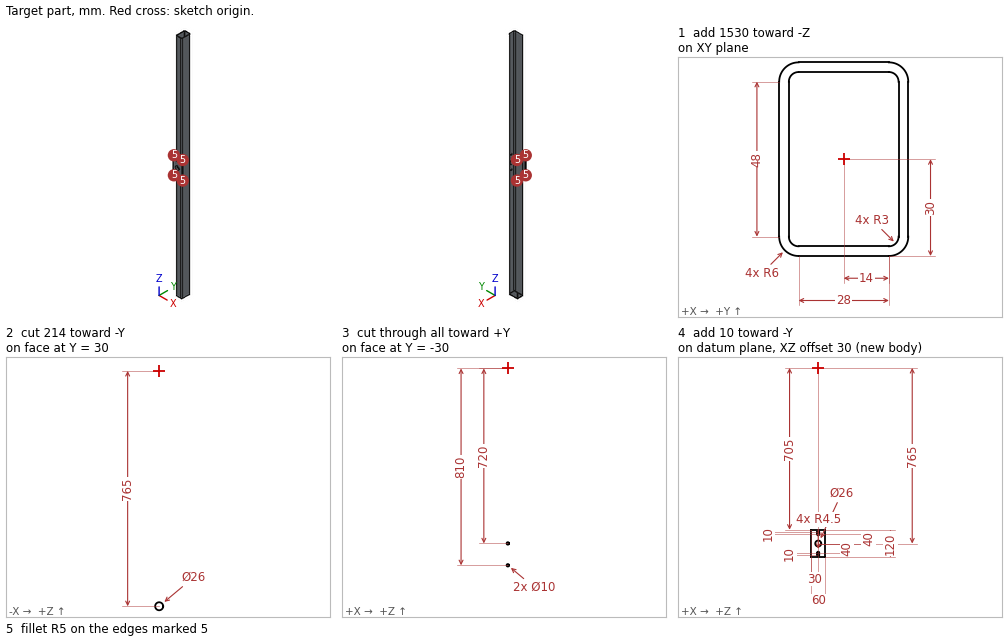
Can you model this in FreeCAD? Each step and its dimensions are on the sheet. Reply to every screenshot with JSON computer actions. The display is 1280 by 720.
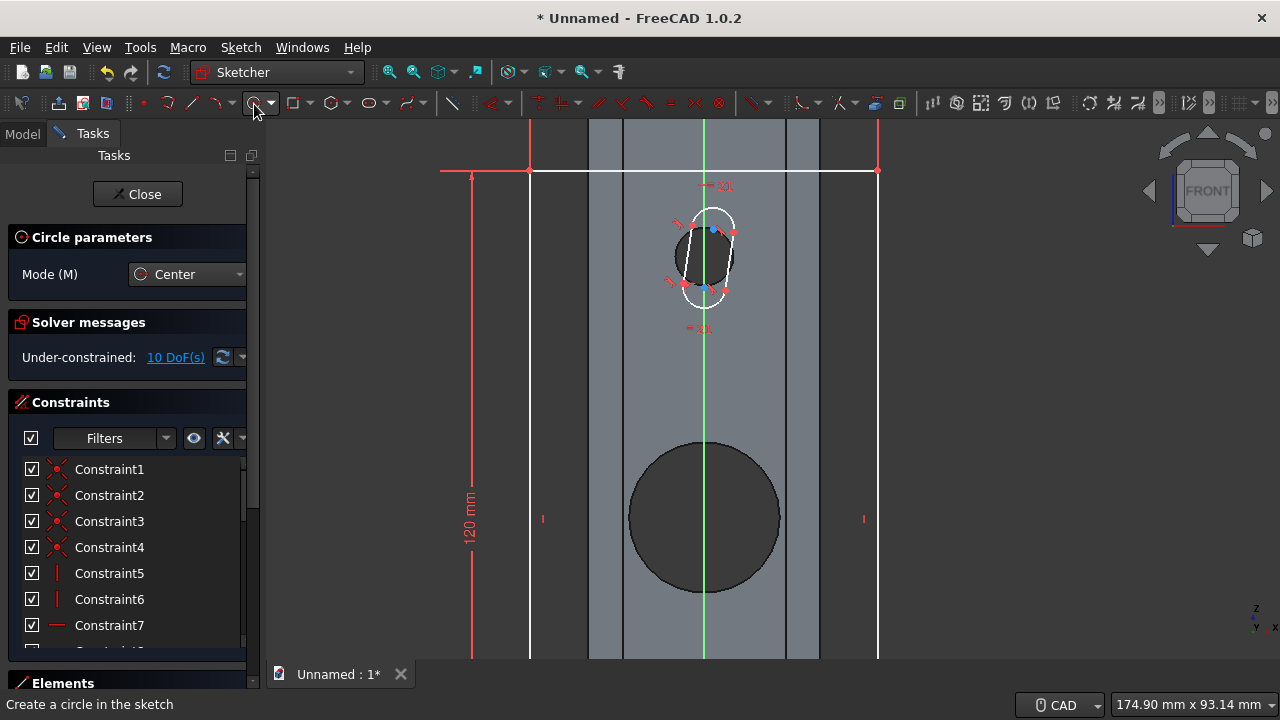
{"action": "left_click", "coordinate": [704, 518]}
{"action": "mouse_move", "coordinate": [758, 464]}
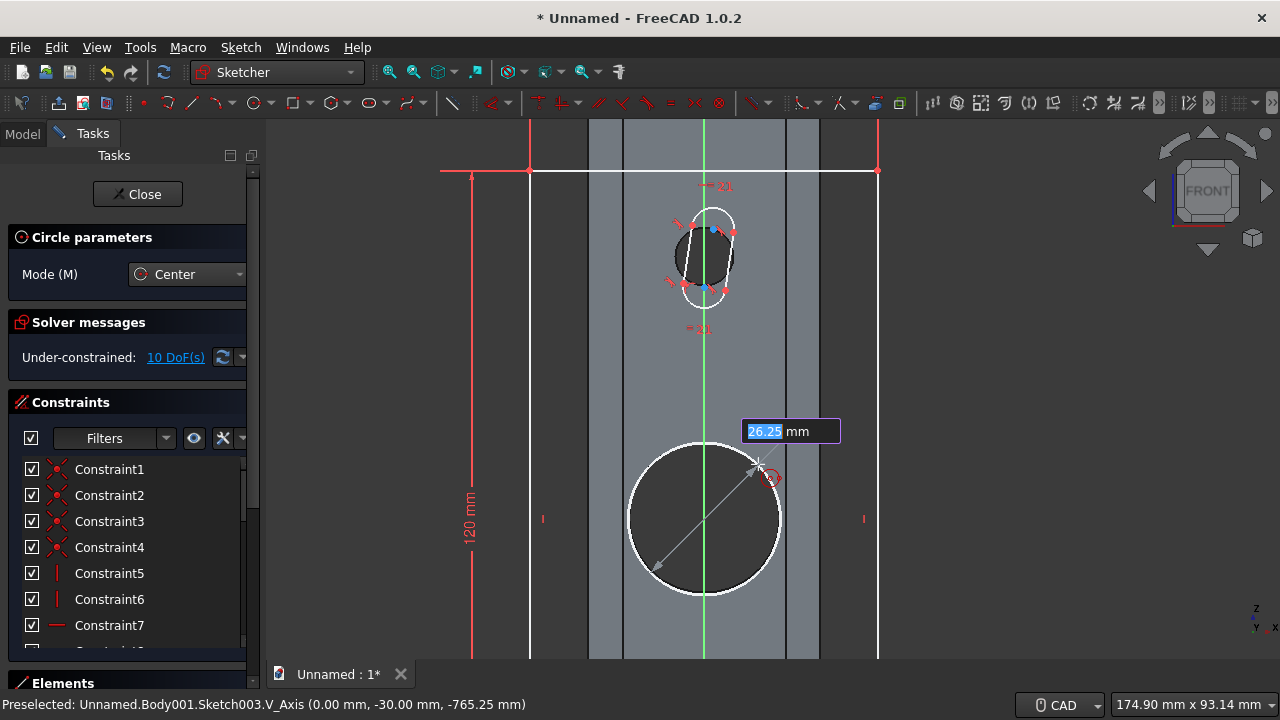
{"action": "type", "text": "26"}
{"action": "key", "text": "Return"}
{"action": "key", "text": "Escape"}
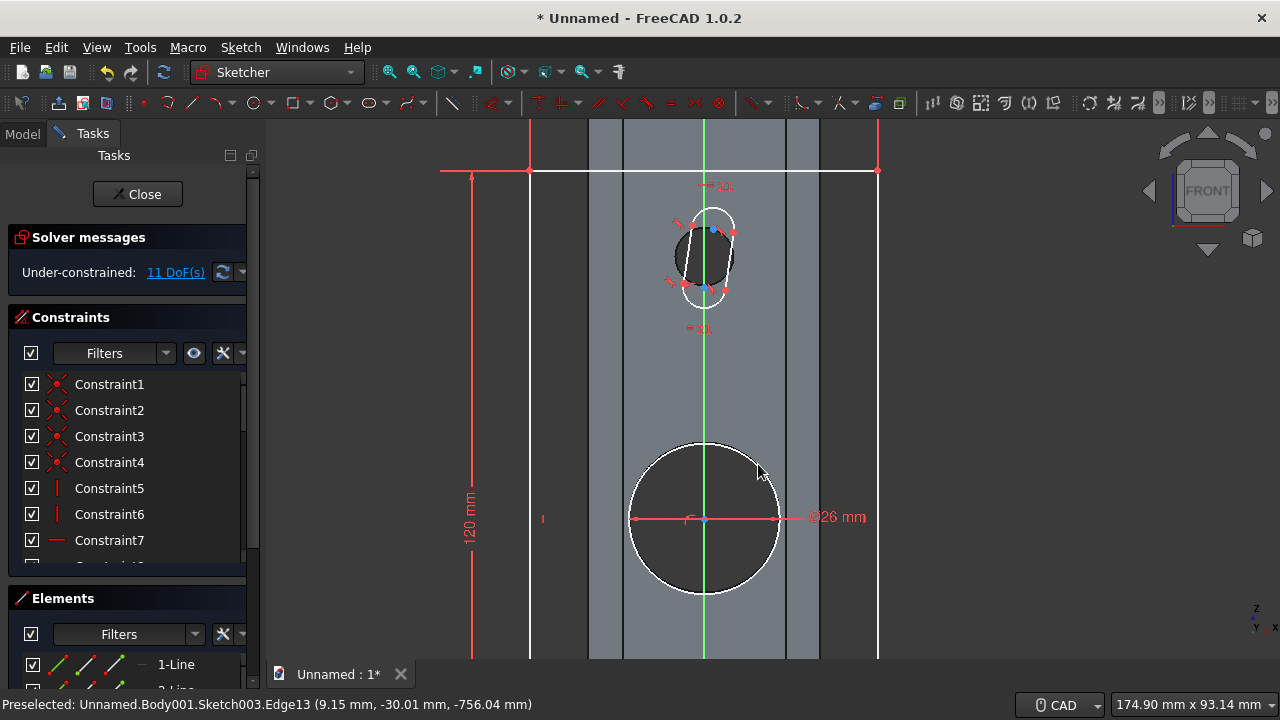
{"action": "scroll", "coordinate": [705, 284], "scroll_direction": "down", "scroll_amount": 4}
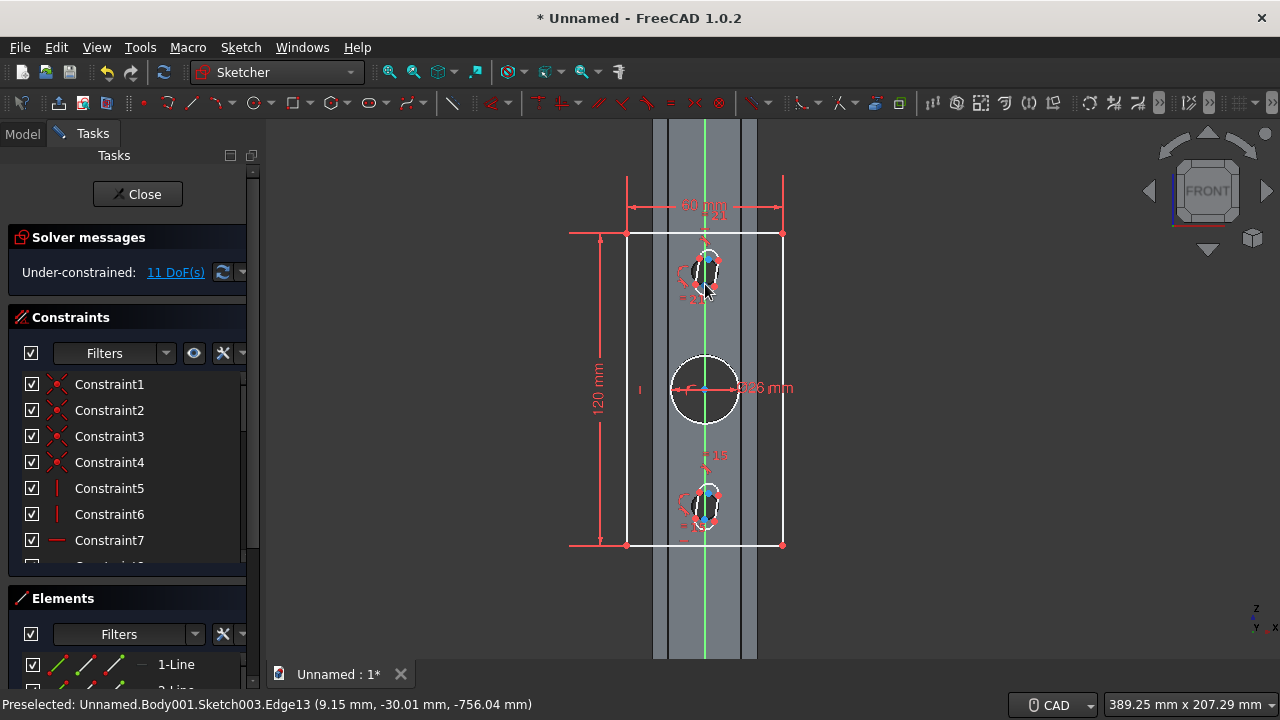
{"action": "scroll", "coordinate": [696, 510], "scroll_direction": "up", "scroll_amount": 3}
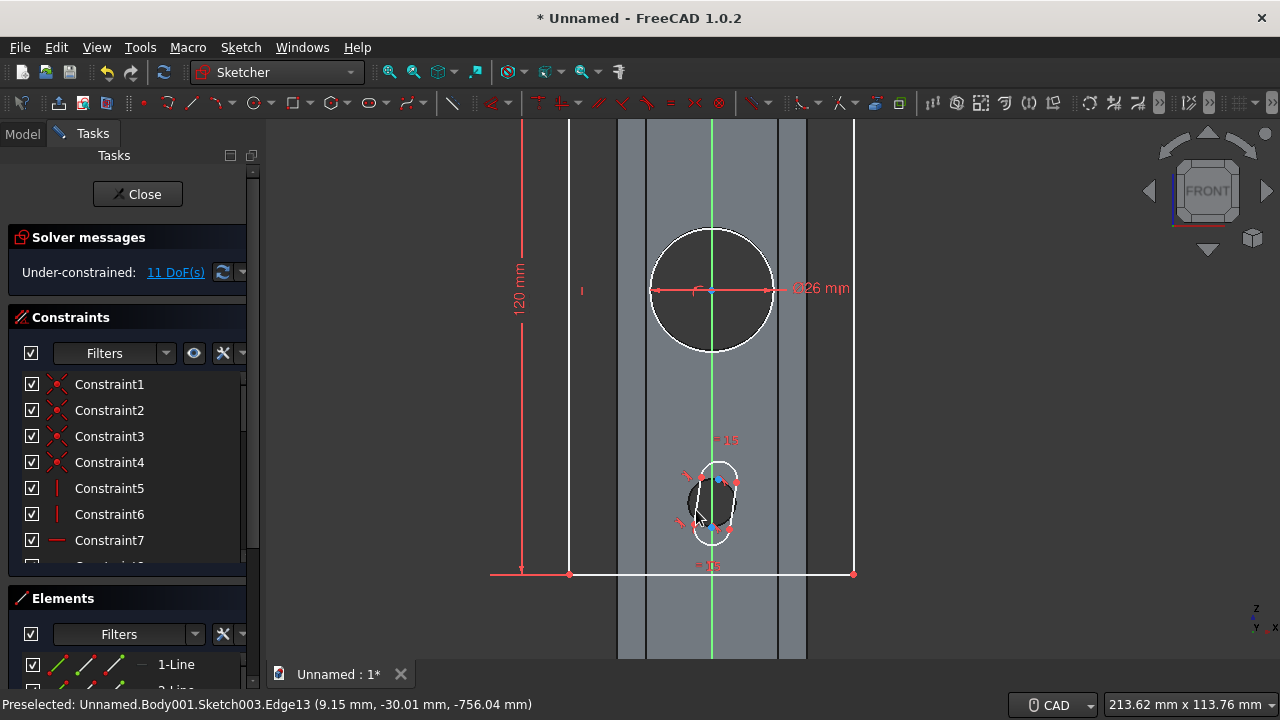
{"action": "left_click", "coordinate": [696, 510]}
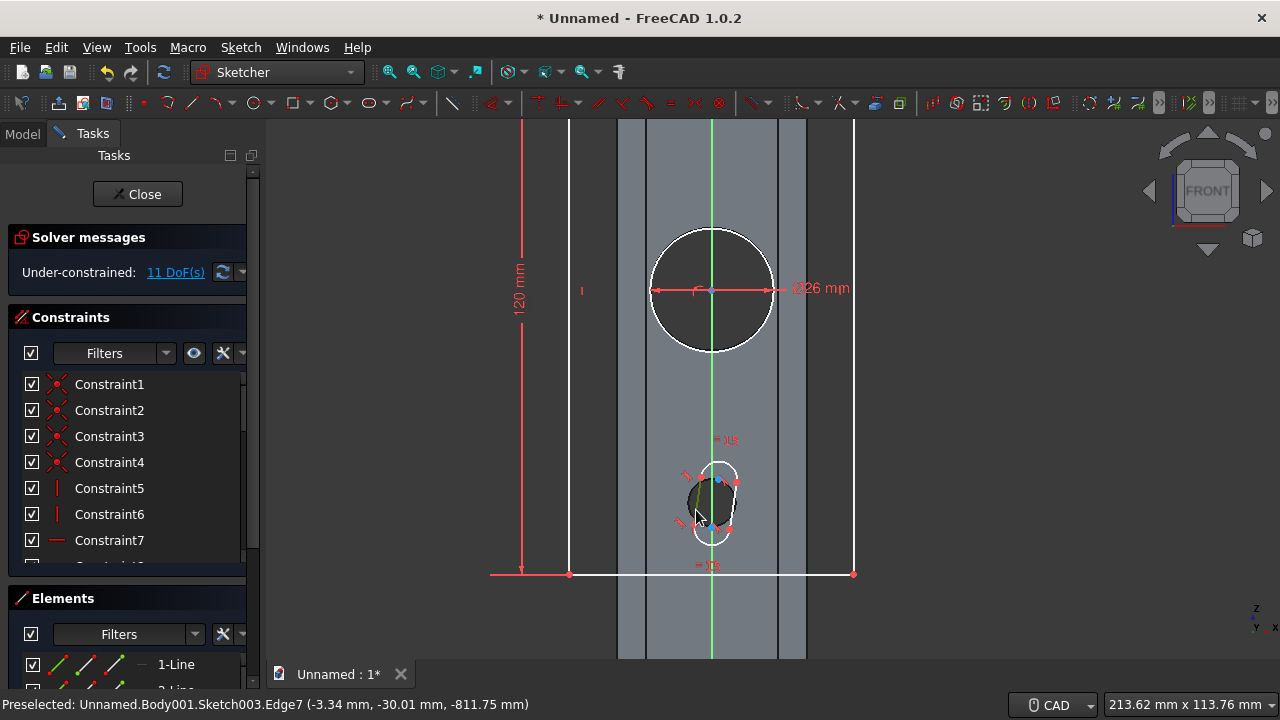
{"action": "key", "text": "v"}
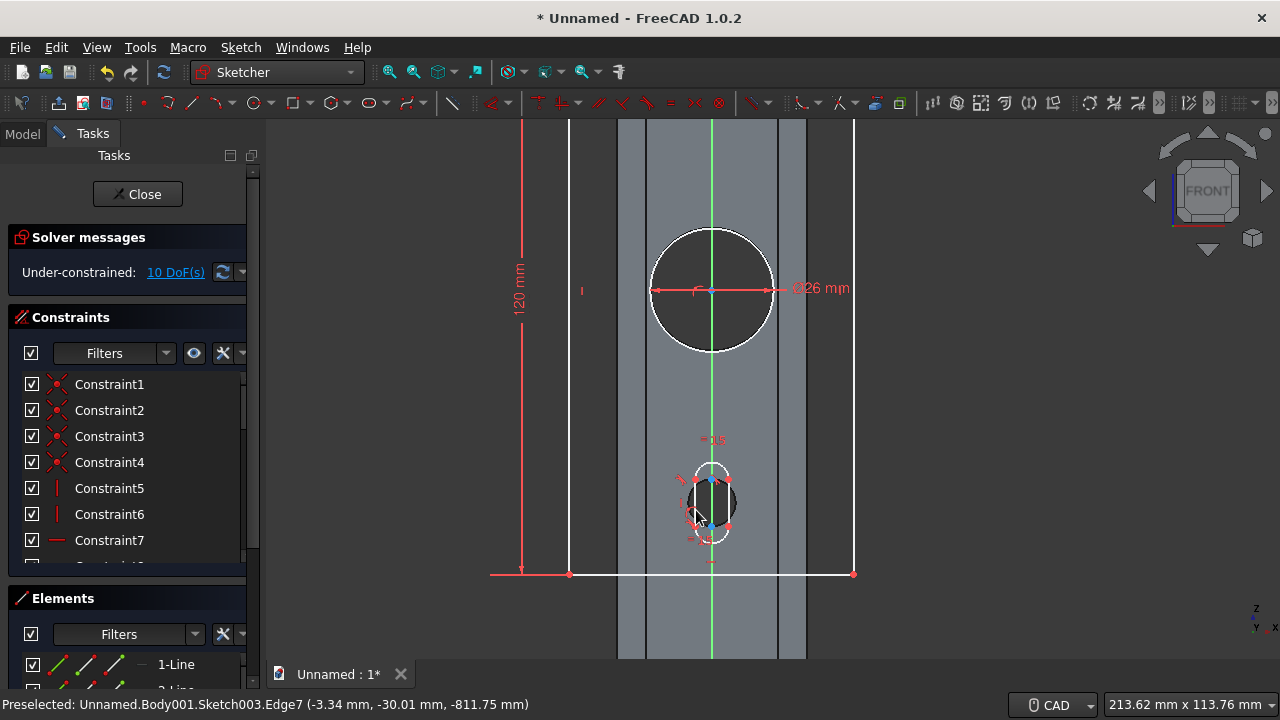
{"action": "scroll", "coordinate": [695, 510], "scroll_direction": "down", "scroll_amount": 3}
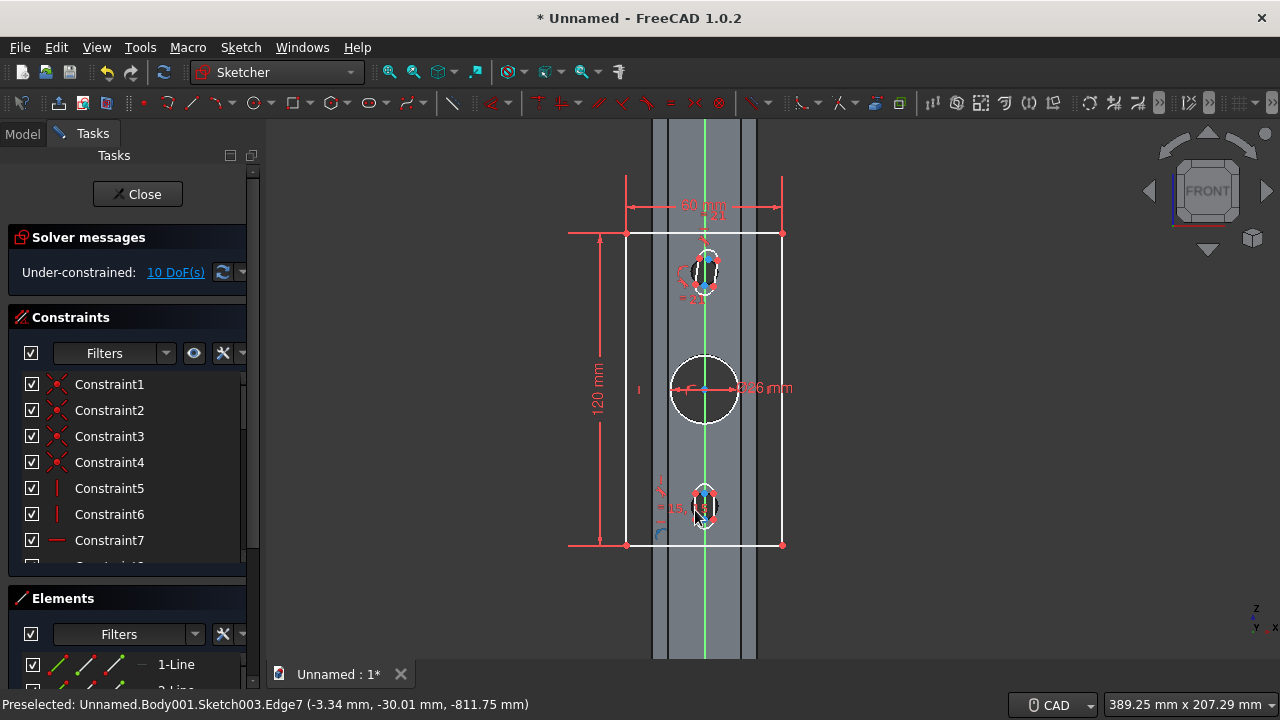
{"action": "scroll", "coordinate": [696, 276], "scroll_direction": "up", "scroll_amount": 3}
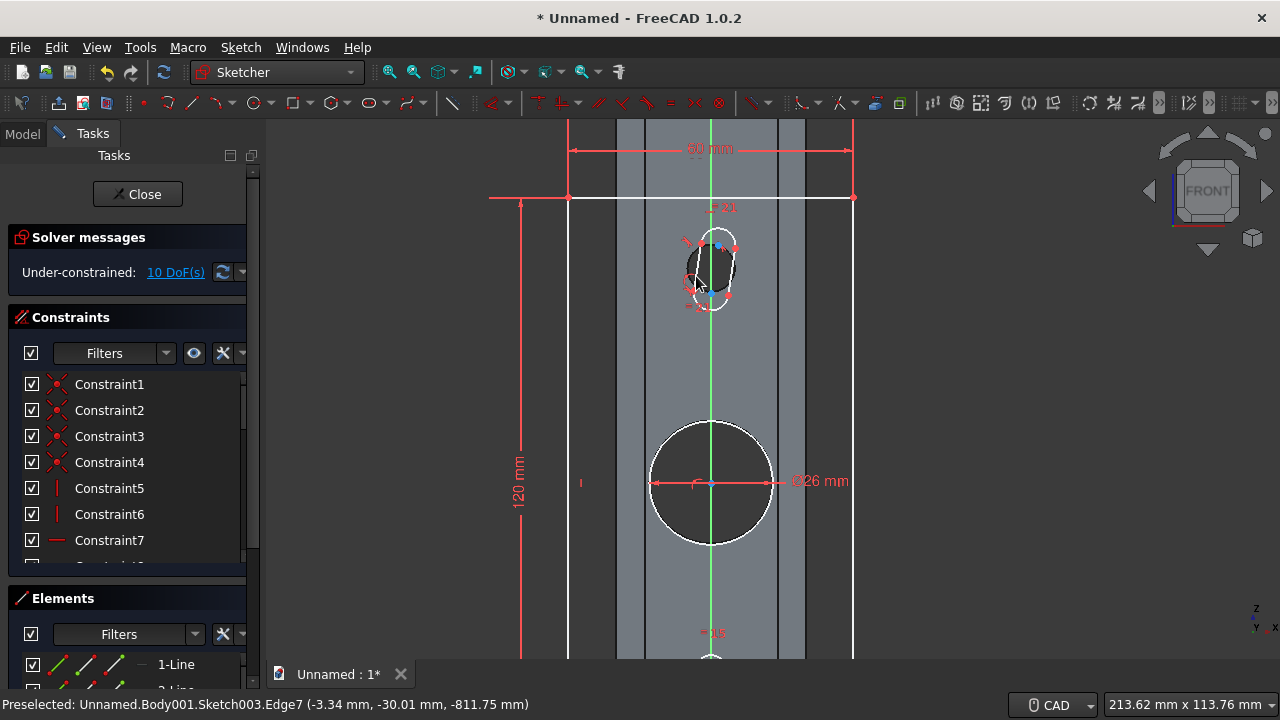
{"action": "left_click", "coordinate": [699, 257]}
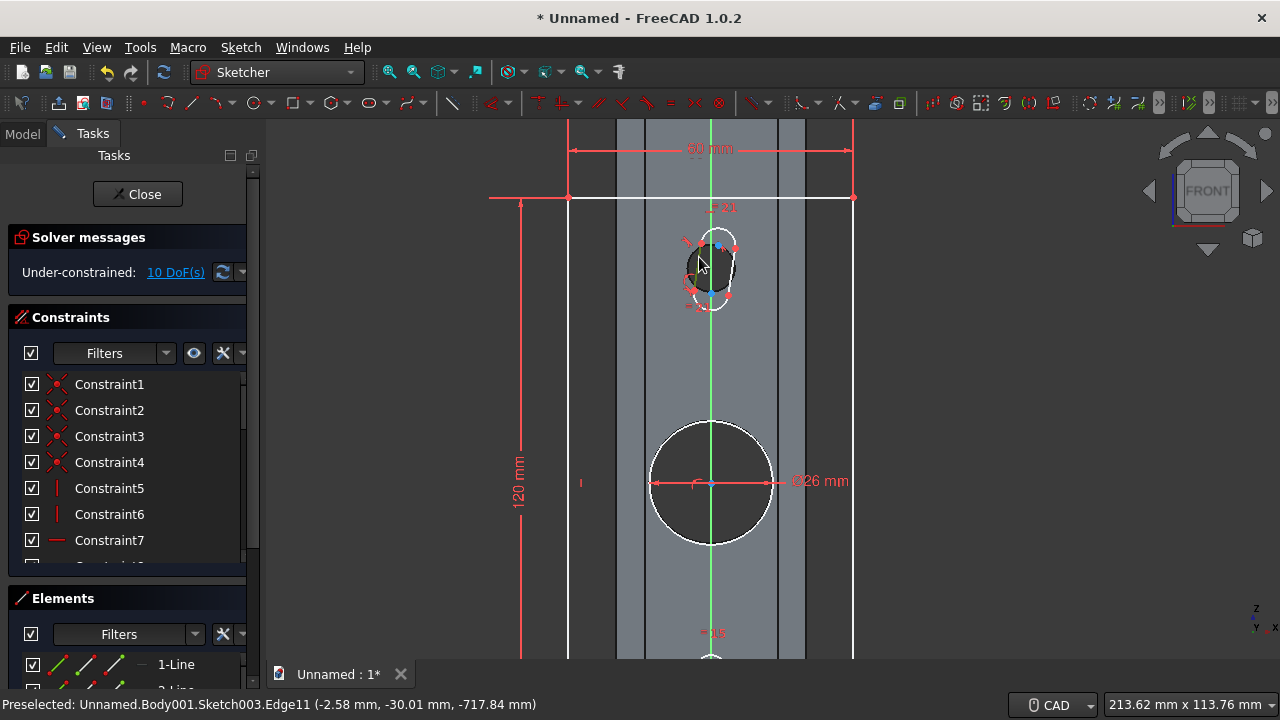
{"action": "left_click", "coordinate": [580, 104]}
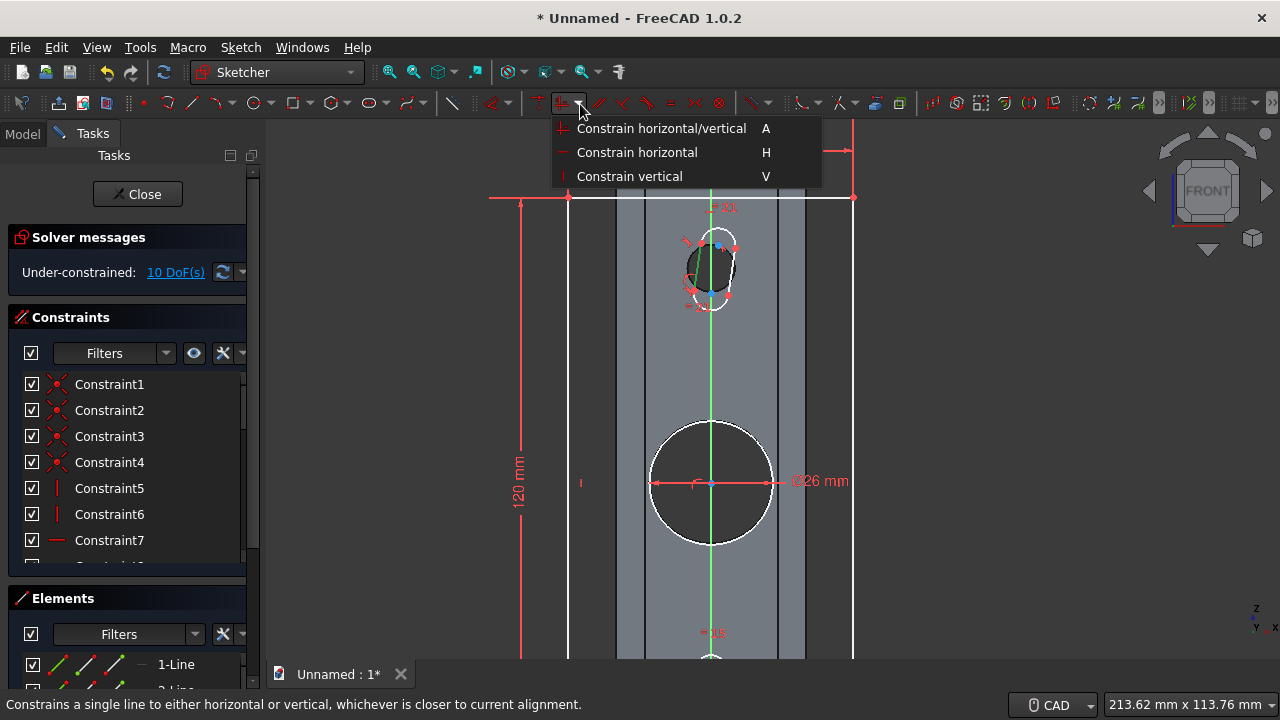
{"action": "left_click", "coordinate": [687, 176]}